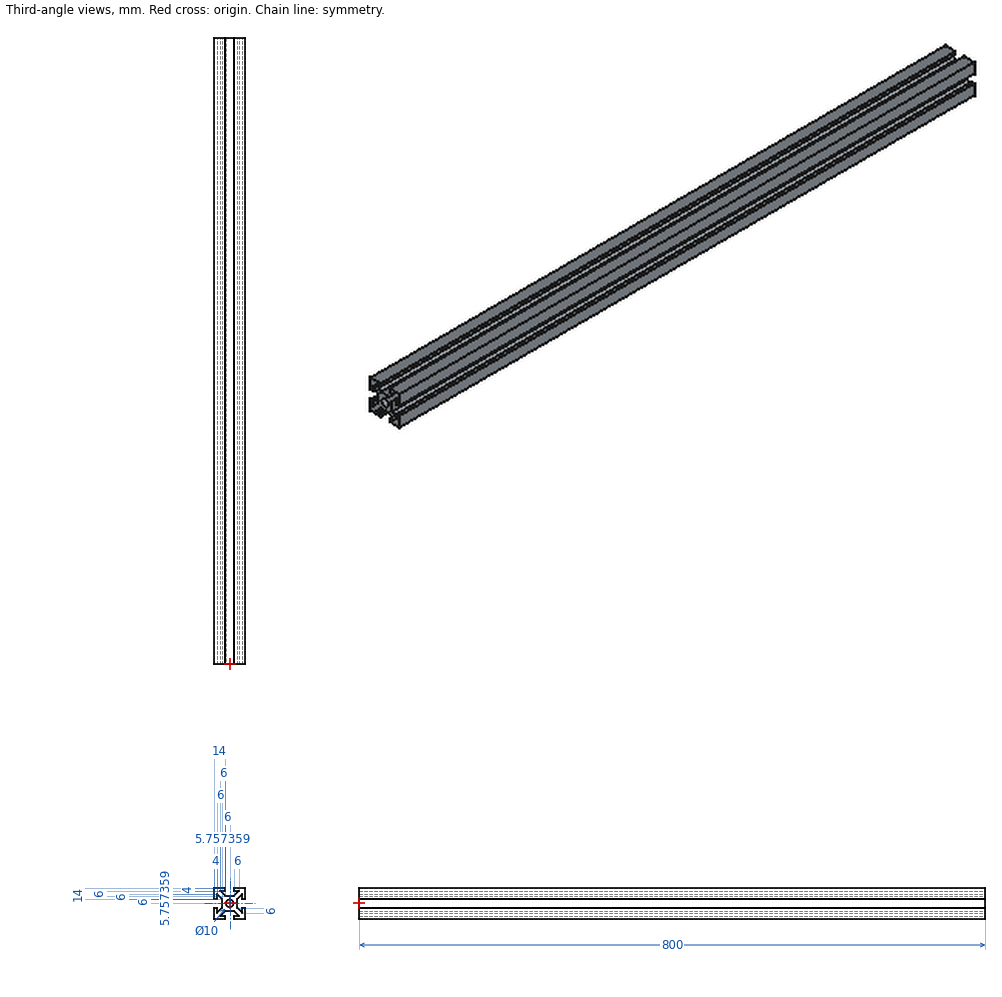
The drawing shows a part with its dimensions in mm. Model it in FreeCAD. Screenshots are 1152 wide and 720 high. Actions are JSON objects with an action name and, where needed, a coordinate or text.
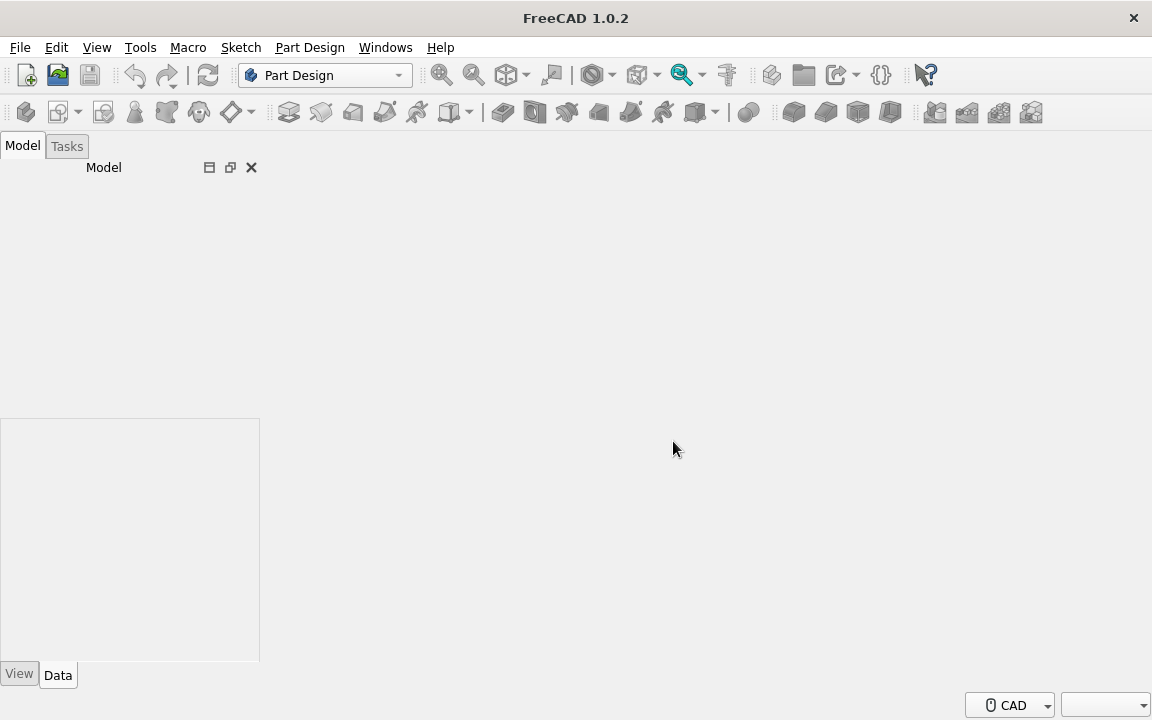
{"action": "key", "text": "ctrl+n"}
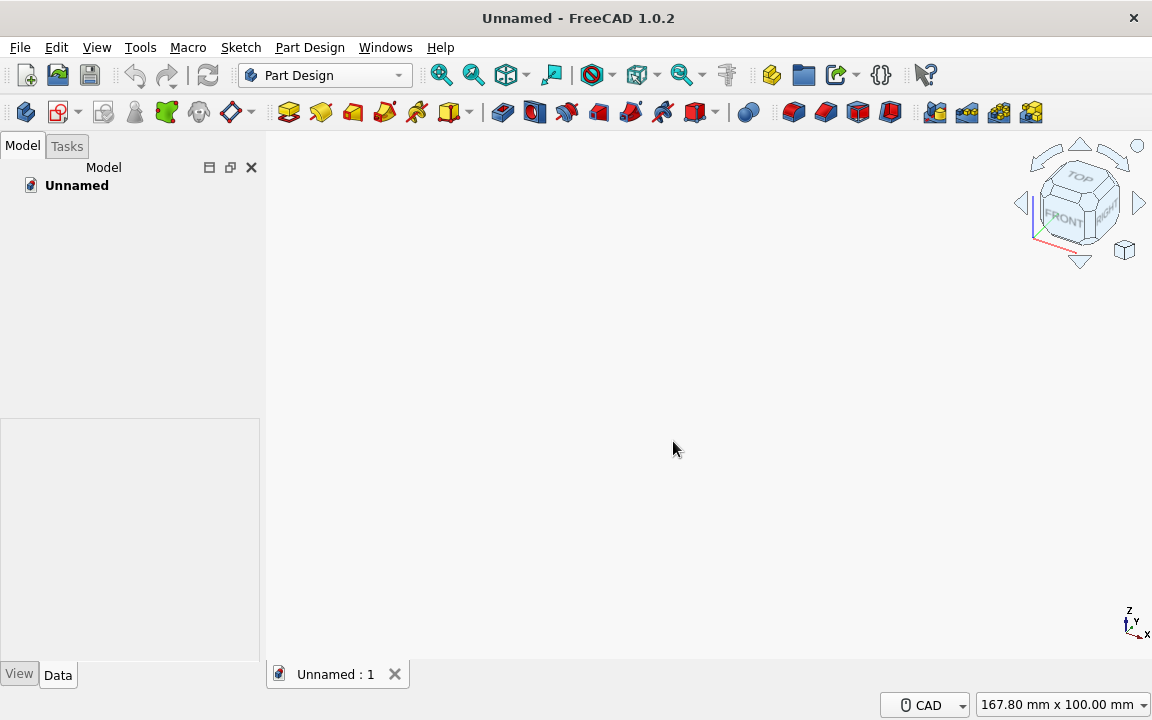
{"action": "left_click", "coordinate": [58, 112]}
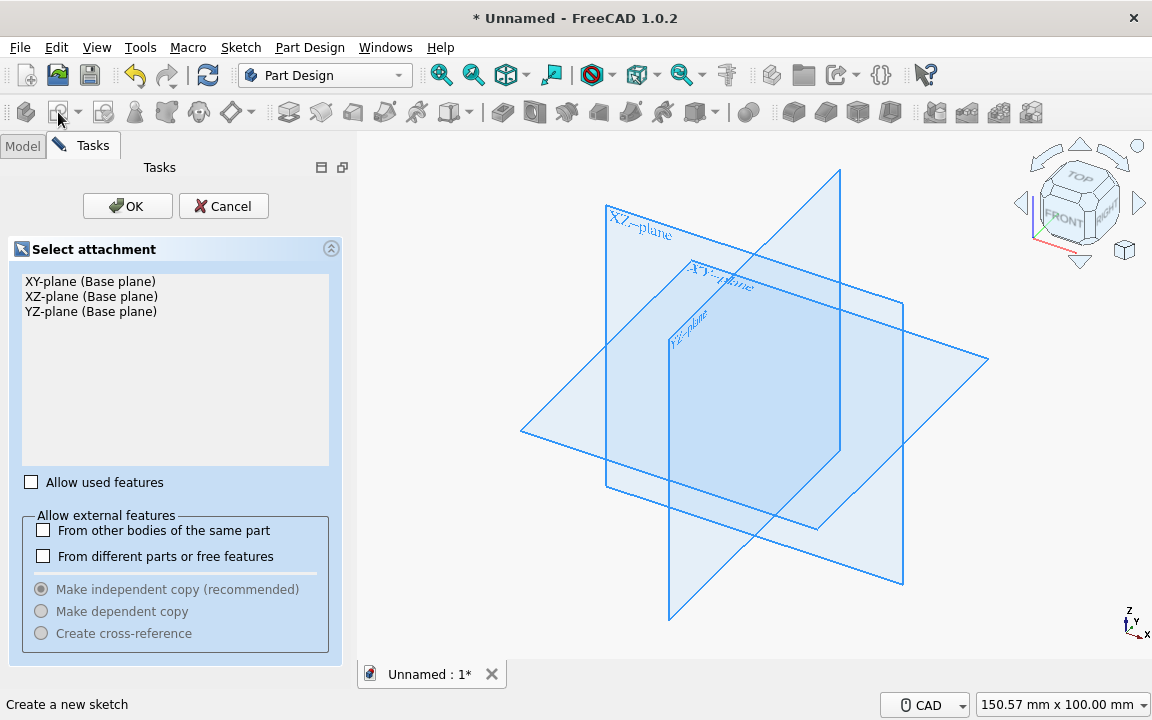
{"action": "left_click", "coordinate": [82, 296]}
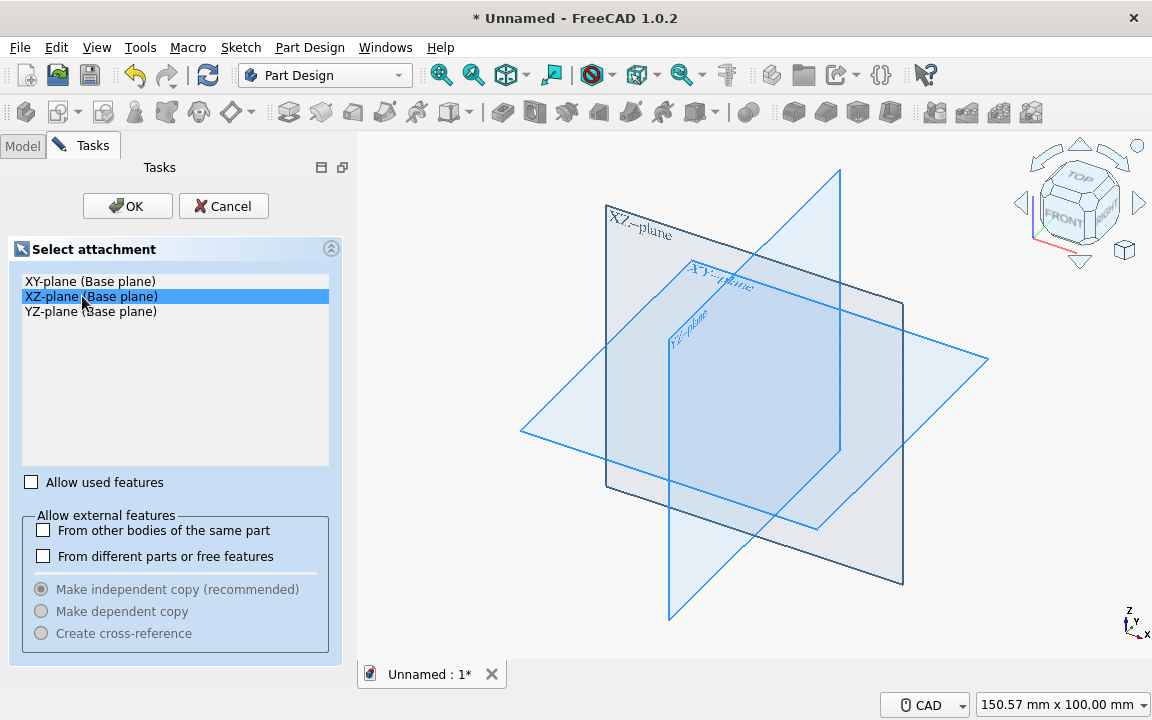
{"action": "left_click", "coordinate": [128, 206]}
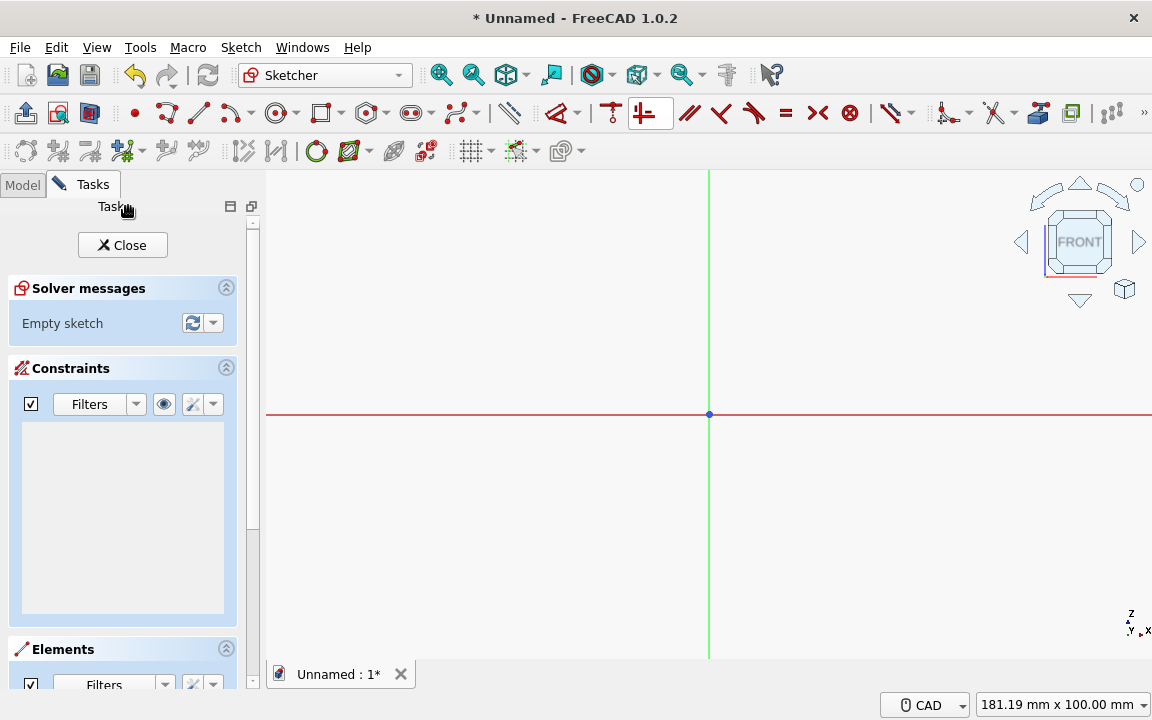
{"action": "scroll", "coordinate": [848, 414], "scroll_direction": "up", "scroll_amount": 2}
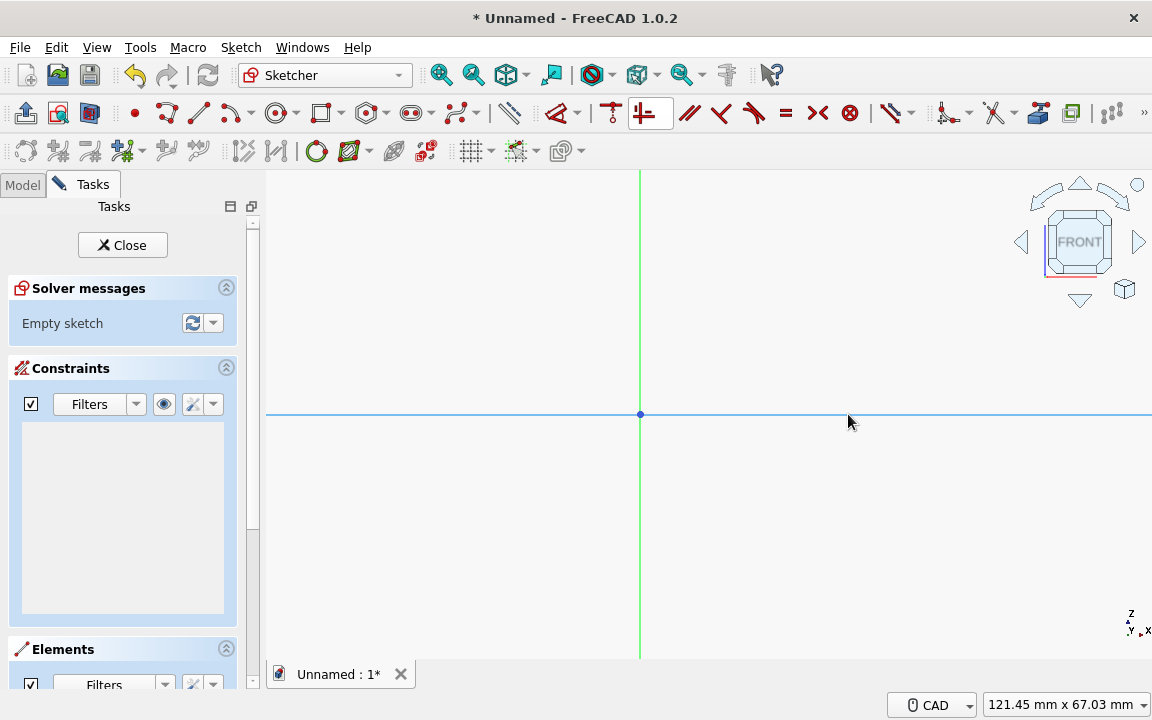
{"action": "left_click", "coordinate": [168, 114]}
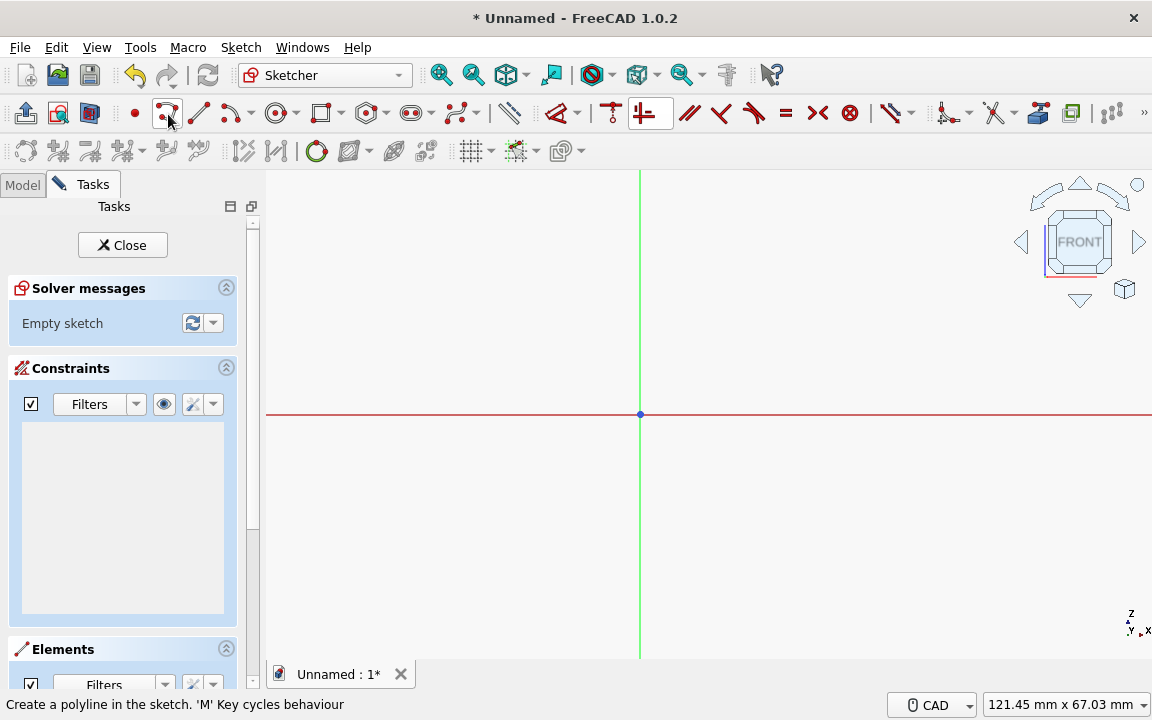
{"action": "left_click", "coordinate": [567, 457]}
{"action": "left_click", "coordinate": [567, 372]}
{"action": "left_click", "coordinate": [524, 329]}
{"action": "left_click", "coordinate": [524, 371]}
{"action": "left_click", "coordinate": [494, 371]}
{"action": "left_click", "coordinate": [494, 269]}
{"action": "left_click", "coordinate": [597, 269]}
{"action": "left_click", "coordinate": [597, 298]}
{"action": "left_click", "coordinate": [555, 298]}
{"action": "left_click", "coordinate": [598, 342]}
{"action": "left_click", "coordinate": [682, 342]}
{"action": "left_click", "coordinate": [726, 298]}
{"action": "left_click", "coordinate": [684, 298]}
{"action": "left_click", "coordinate": [684, 269]}
{"action": "left_click", "coordinate": [786, 269]}
{"action": "left_click", "coordinate": [786, 371]}
{"action": "left_click", "coordinate": [757, 371]}
{"action": "left_click", "coordinate": [757, 329]}
{"action": "left_click", "coordinate": [713, 372]}
{"action": "left_click", "coordinate": [713, 457]}
{"action": "left_click", "coordinate": [757, 500]}
{"action": "left_click", "coordinate": [757, 458]}
{"action": "left_click", "coordinate": [786, 458]}
{"action": "left_click", "coordinate": [786, 560]}
{"action": "left_click", "coordinate": [684, 560]}
{"action": "left_click", "coordinate": [684, 531]}
{"action": "left_click", "coordinate": [726, 531]}
{"action": "left_click", "coordinate": [682, 487]}
{"action": "left_click", "coordinate": [598, 487]}
{"action": "left_click", "coordinate": [555, 531]}
{"action": "left_click", "coordinate": [597, 531]}
{"action": "left_click", "coordinate": [597, 560]}
{"action": "left_click", "coordinate": [494, 560]}
{"action": "left_click", "coordinate": [494, 458]}
{"action": "left_click", "coordinate": [524, 458]}
{"action": "left_click", "coordinate": [524, 500]}
{"action": "left_click", "coordinate": [567, 458]}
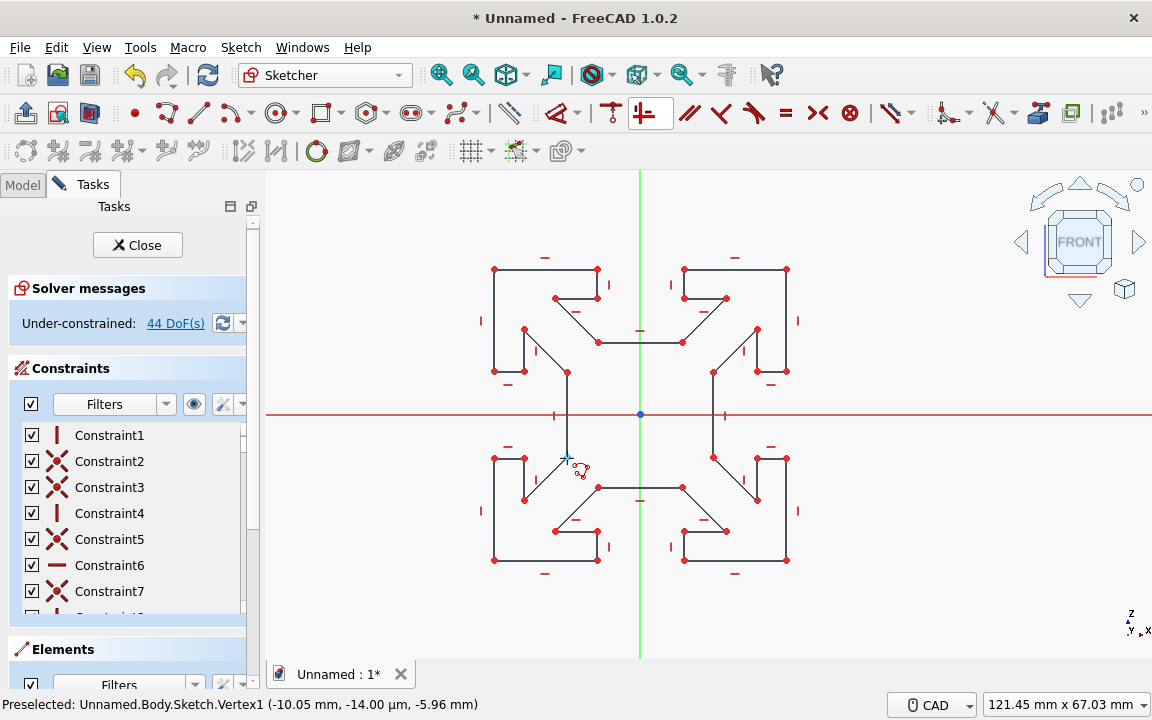
{"action": "left_click", "coordinate": [276, 114]}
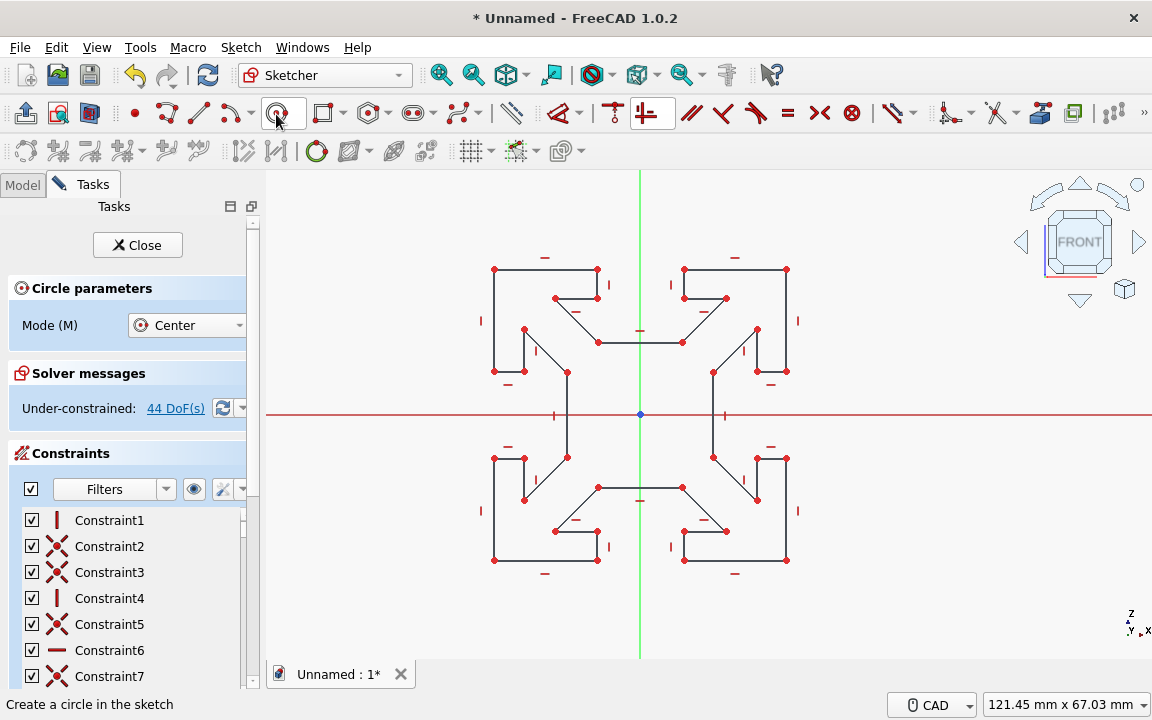
{"action": "left_click", "coordinate": [640, 414]}
{"action": "mouse_move", "coordinate": [666, 389]}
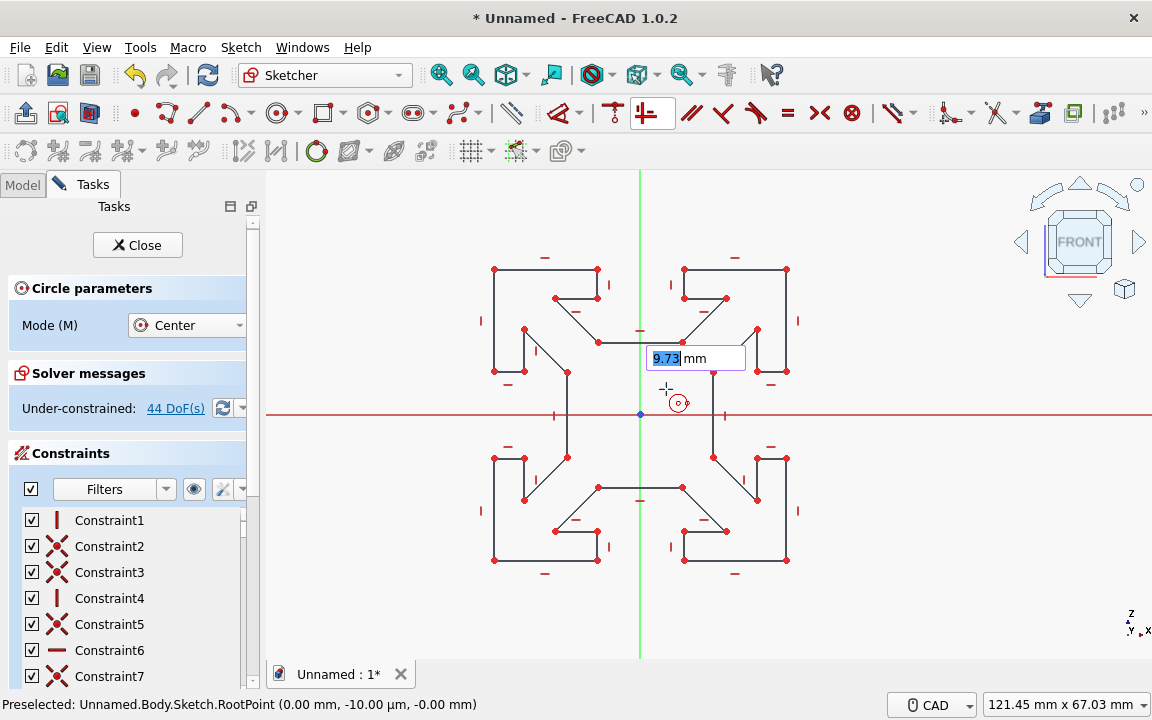
{"action": "type", "text": "10"}
{"action": "key", "text": "Return"}
{"action": "key", "text": "Escape"}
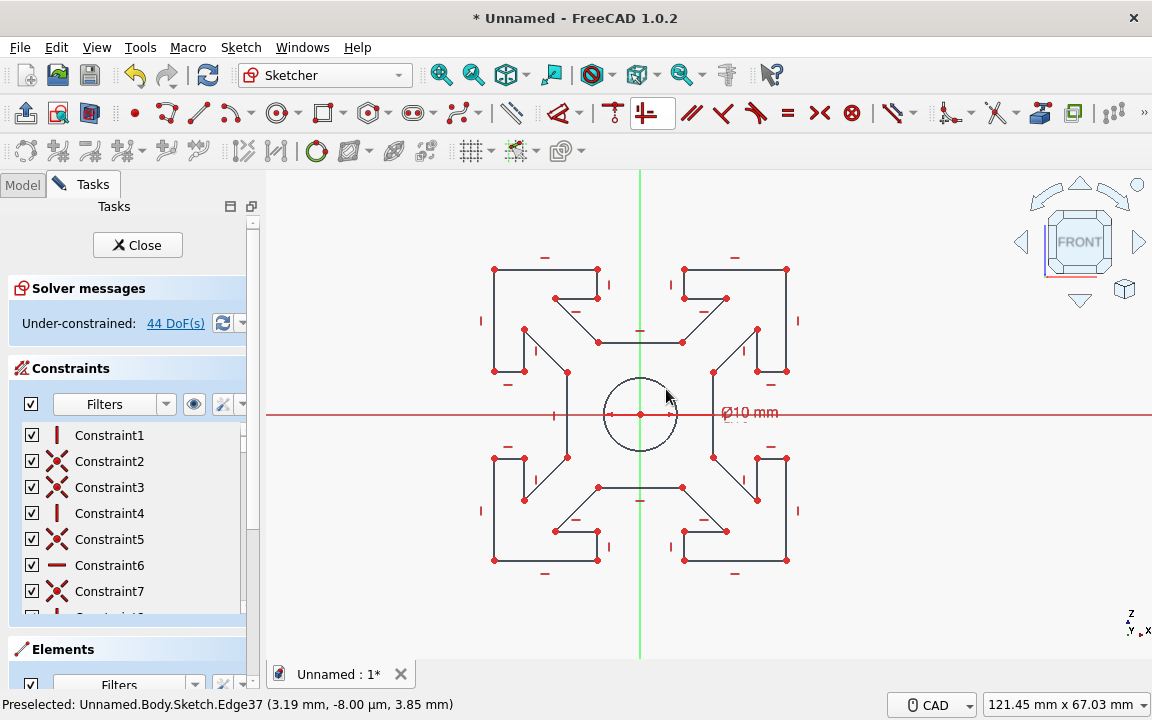
{"action": "left_click", "coordinate": [555, 299]}